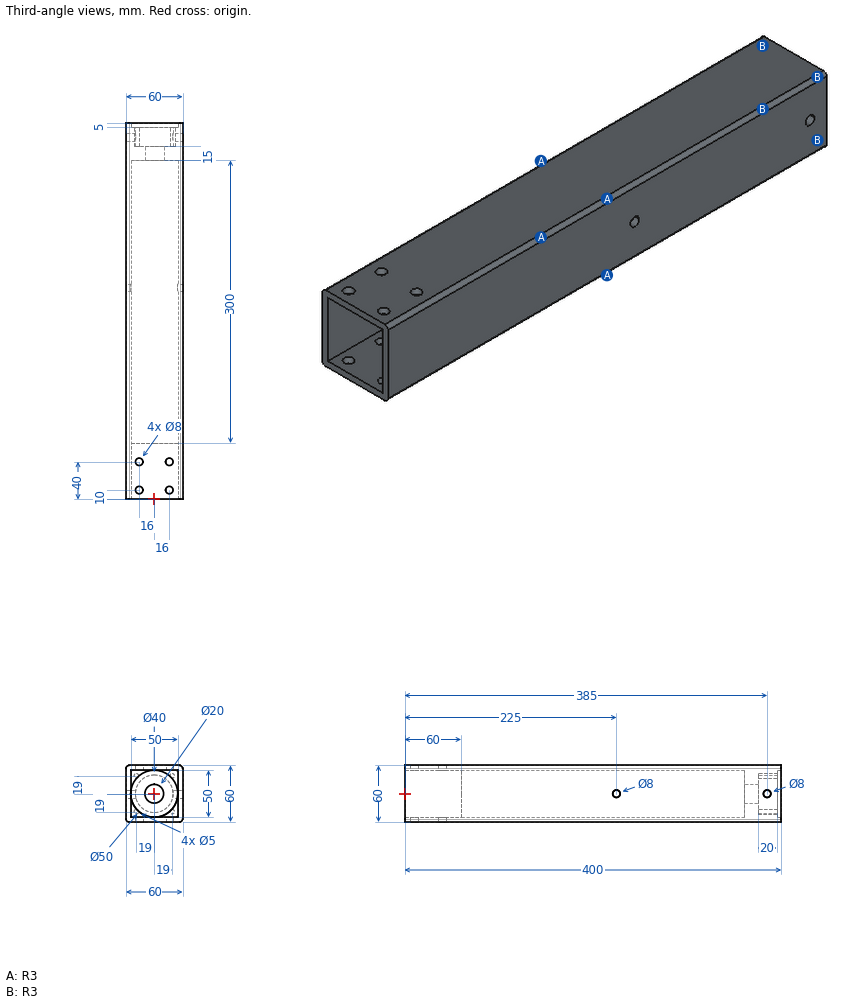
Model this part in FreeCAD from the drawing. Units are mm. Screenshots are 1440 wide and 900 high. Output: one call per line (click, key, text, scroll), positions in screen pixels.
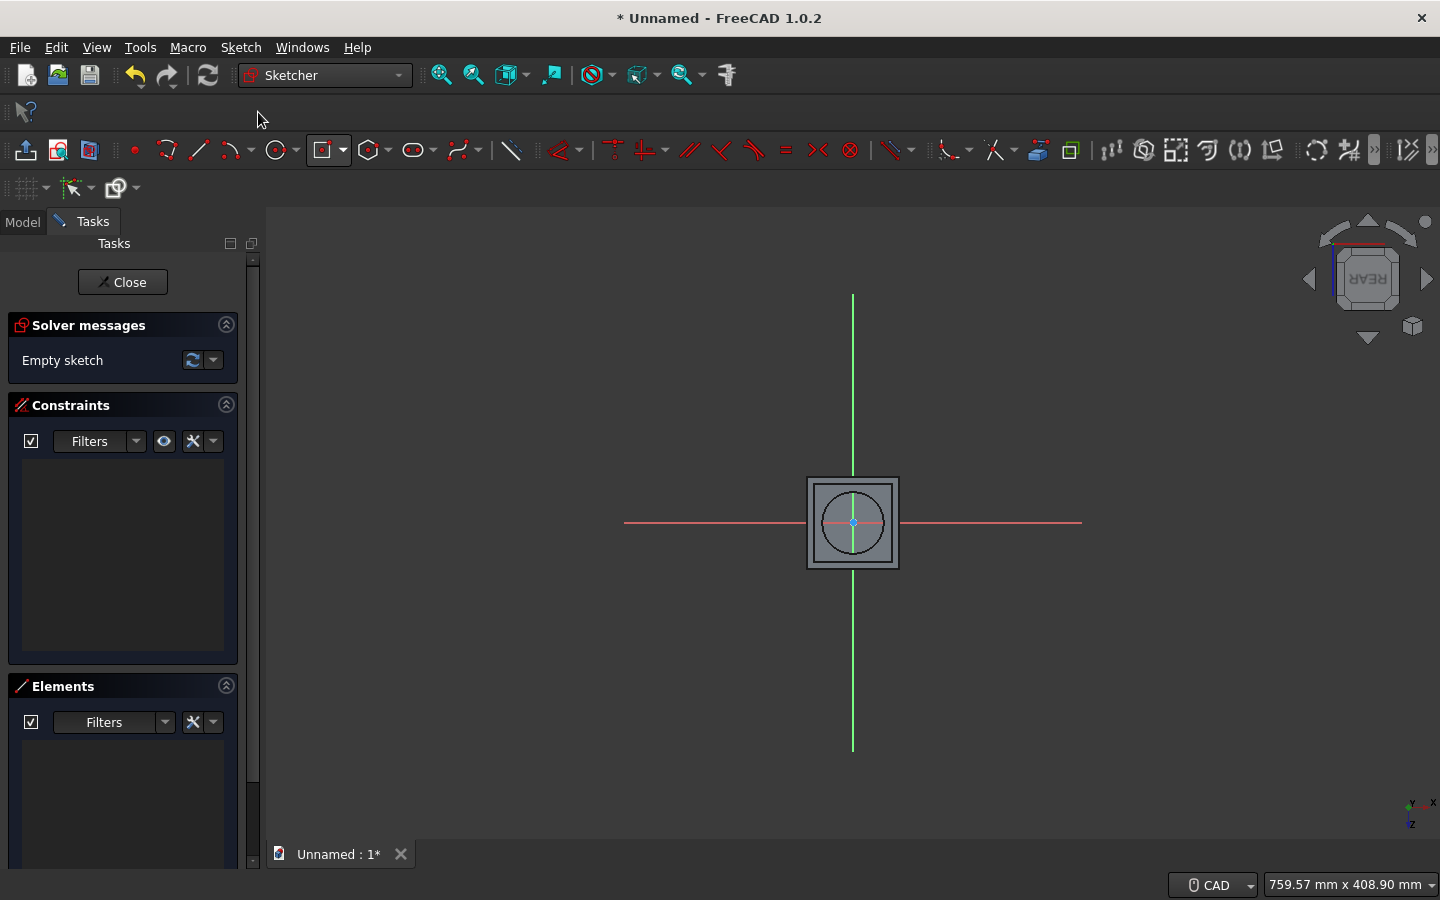
scroll(858, 523, up, 13)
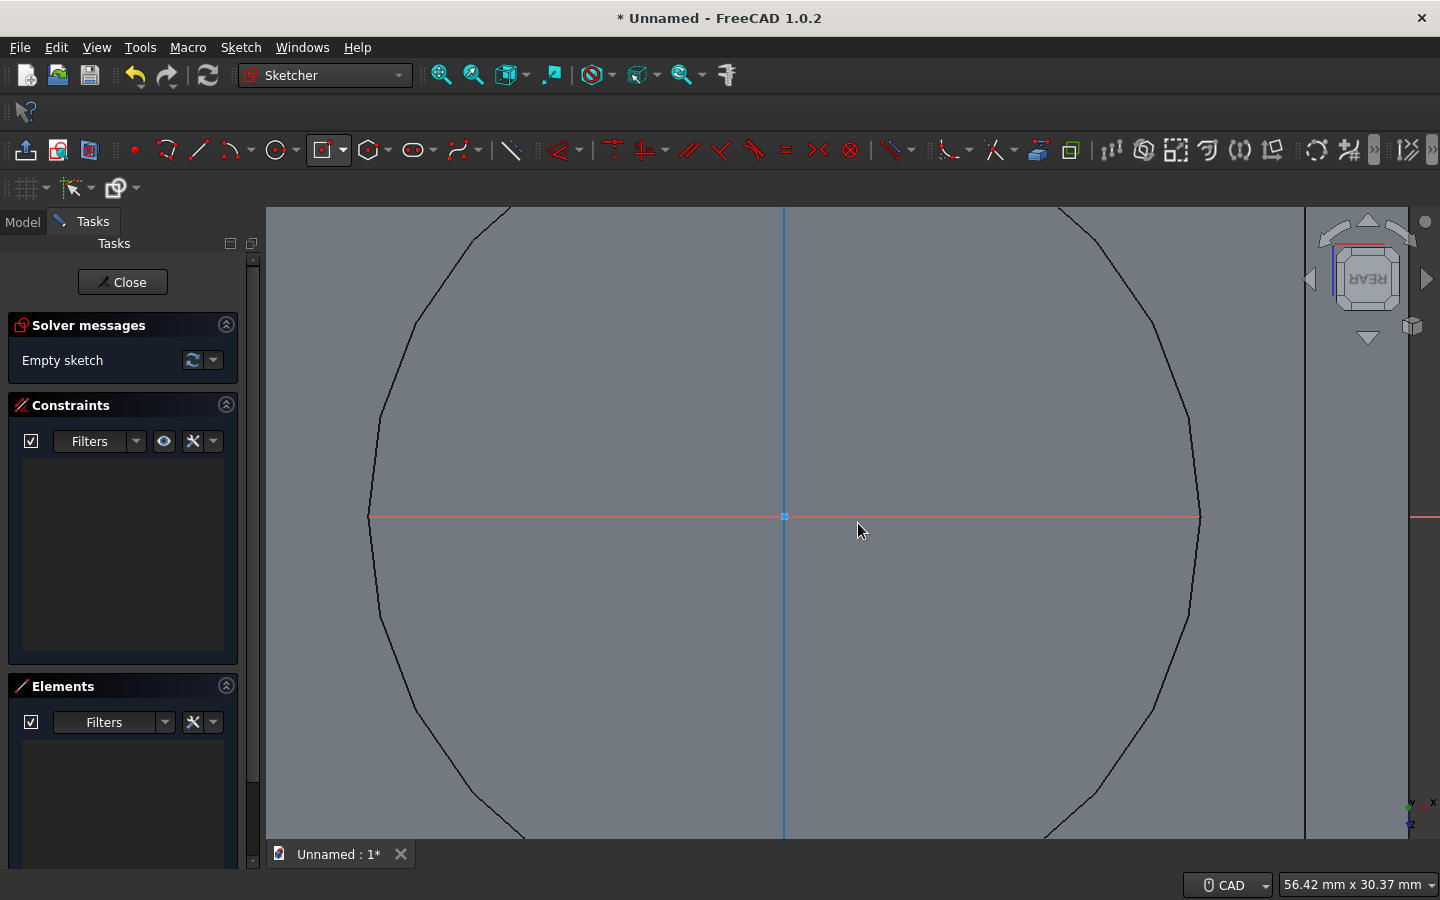
key(g)
key(c)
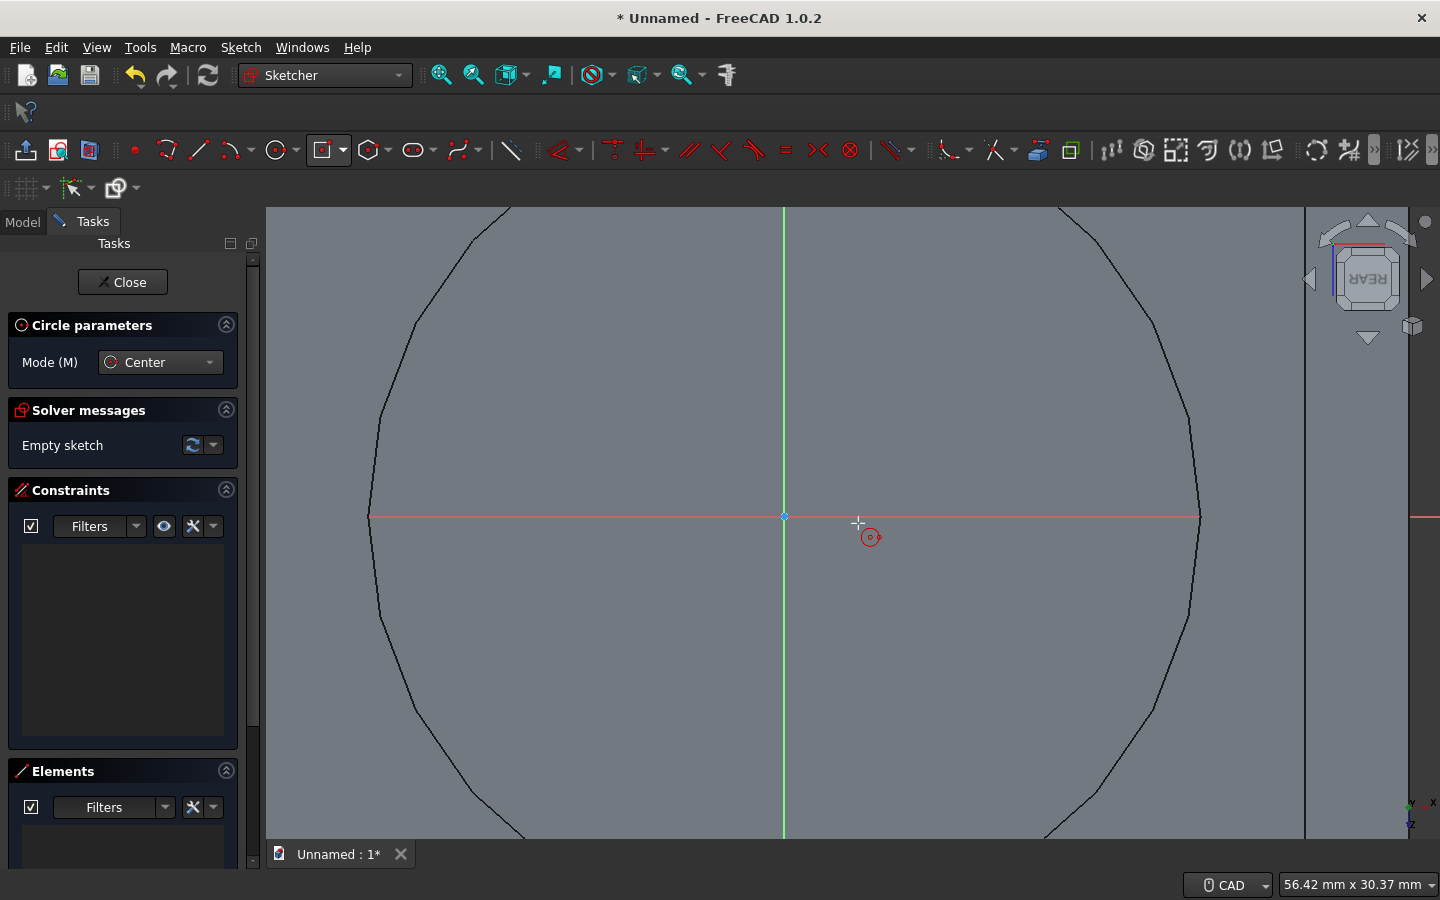
click(784, 517)
move(932, 370)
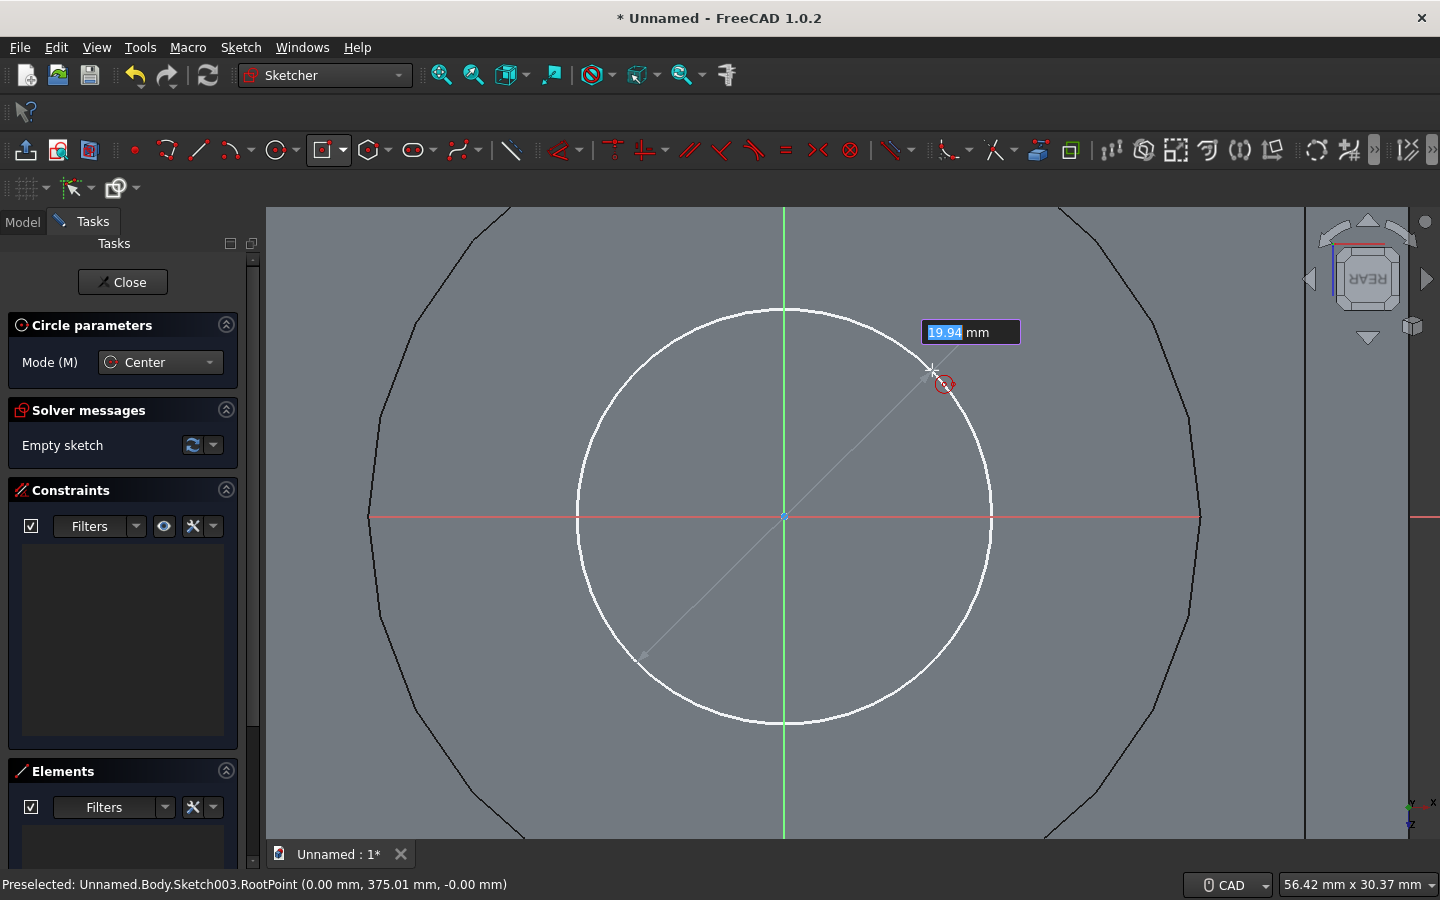
text(20)
key(Return)
key(Escape)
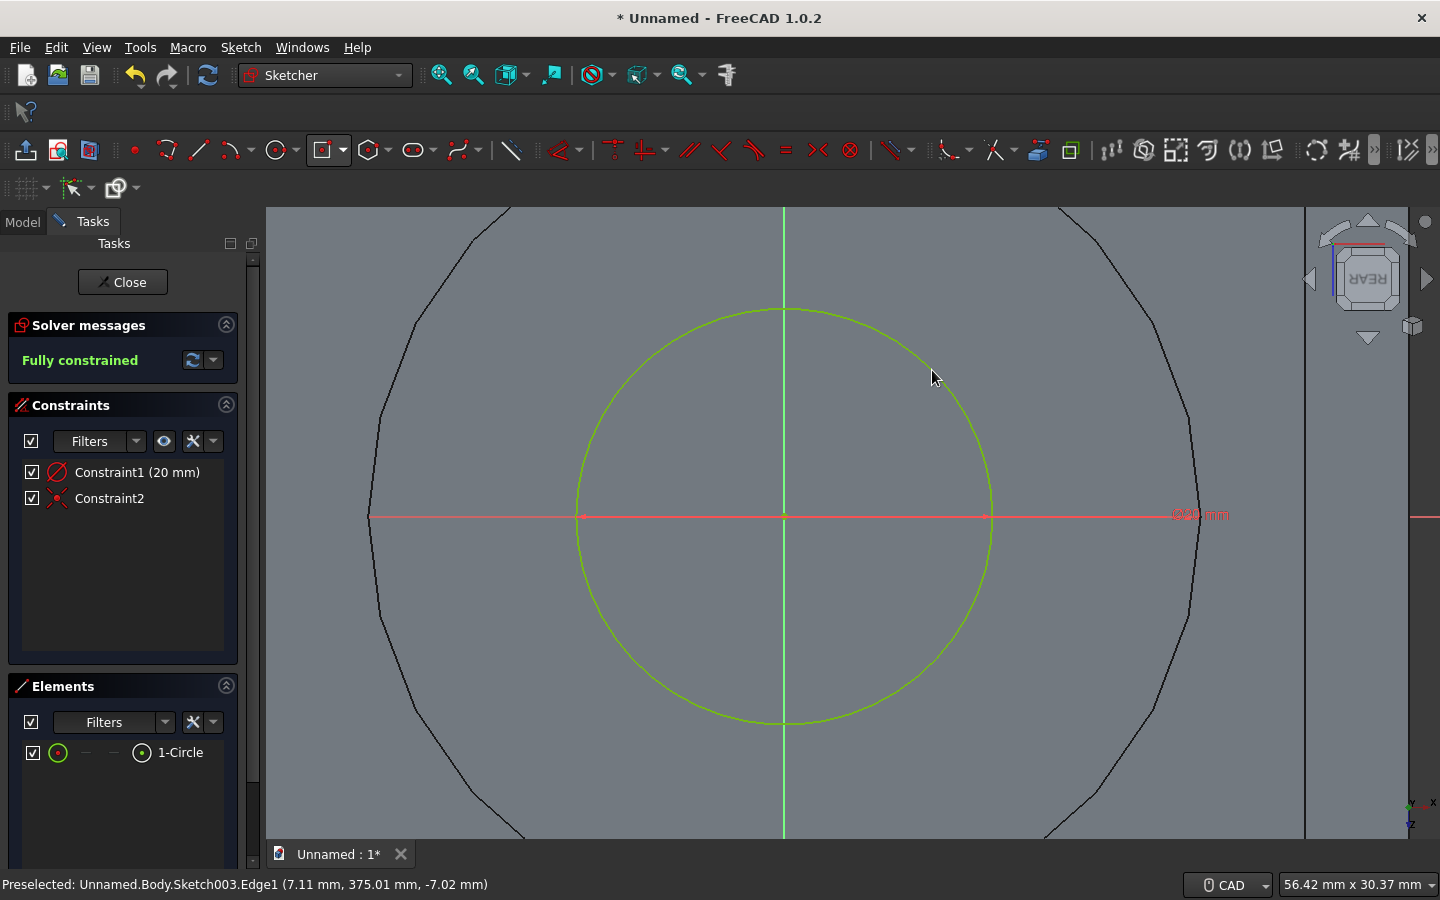
click(123, 282)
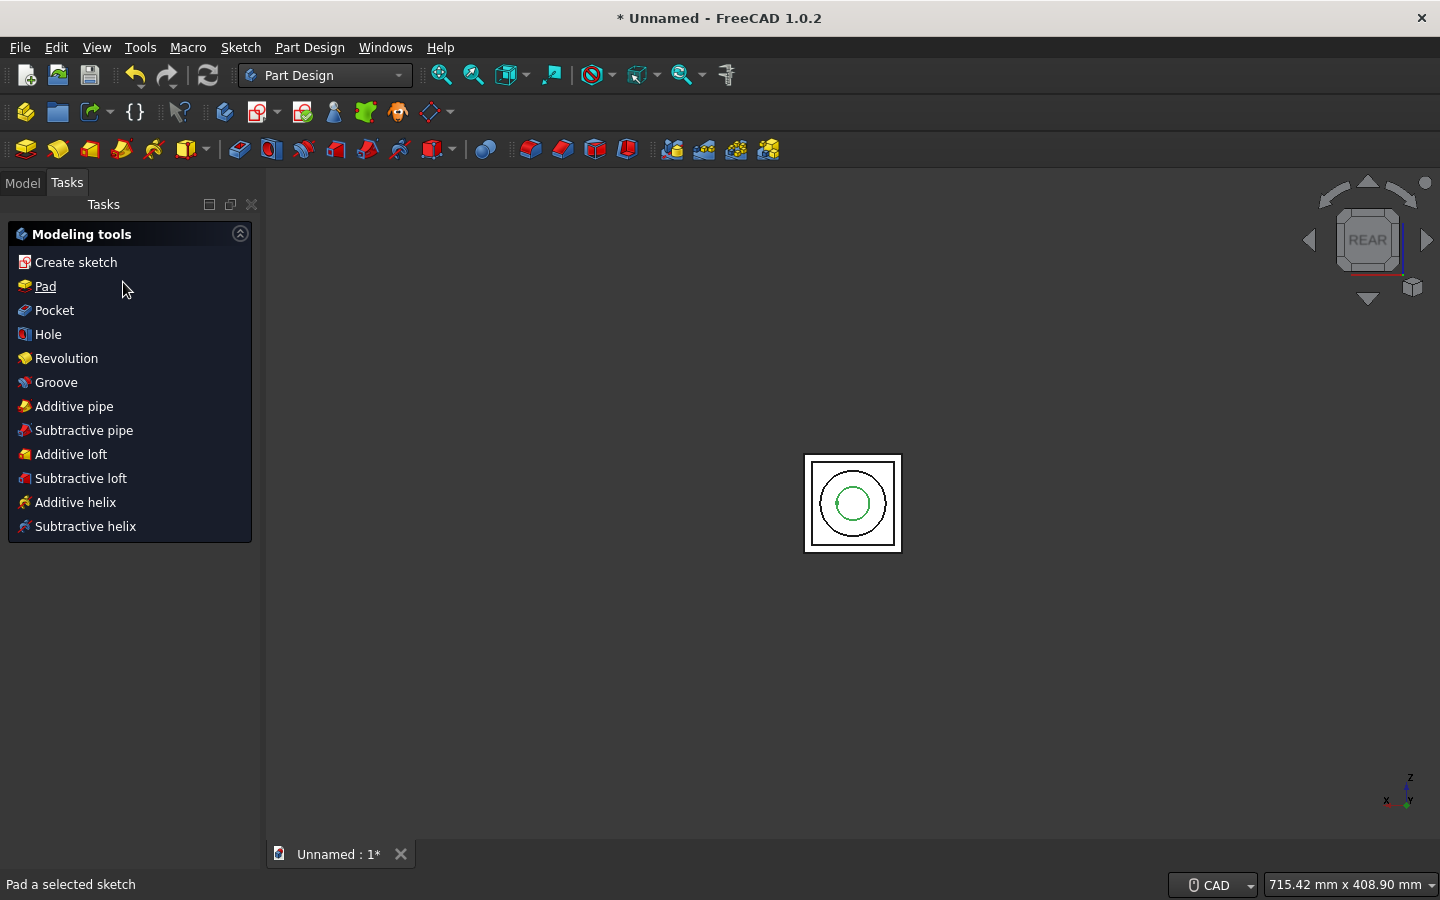
click(240, 150)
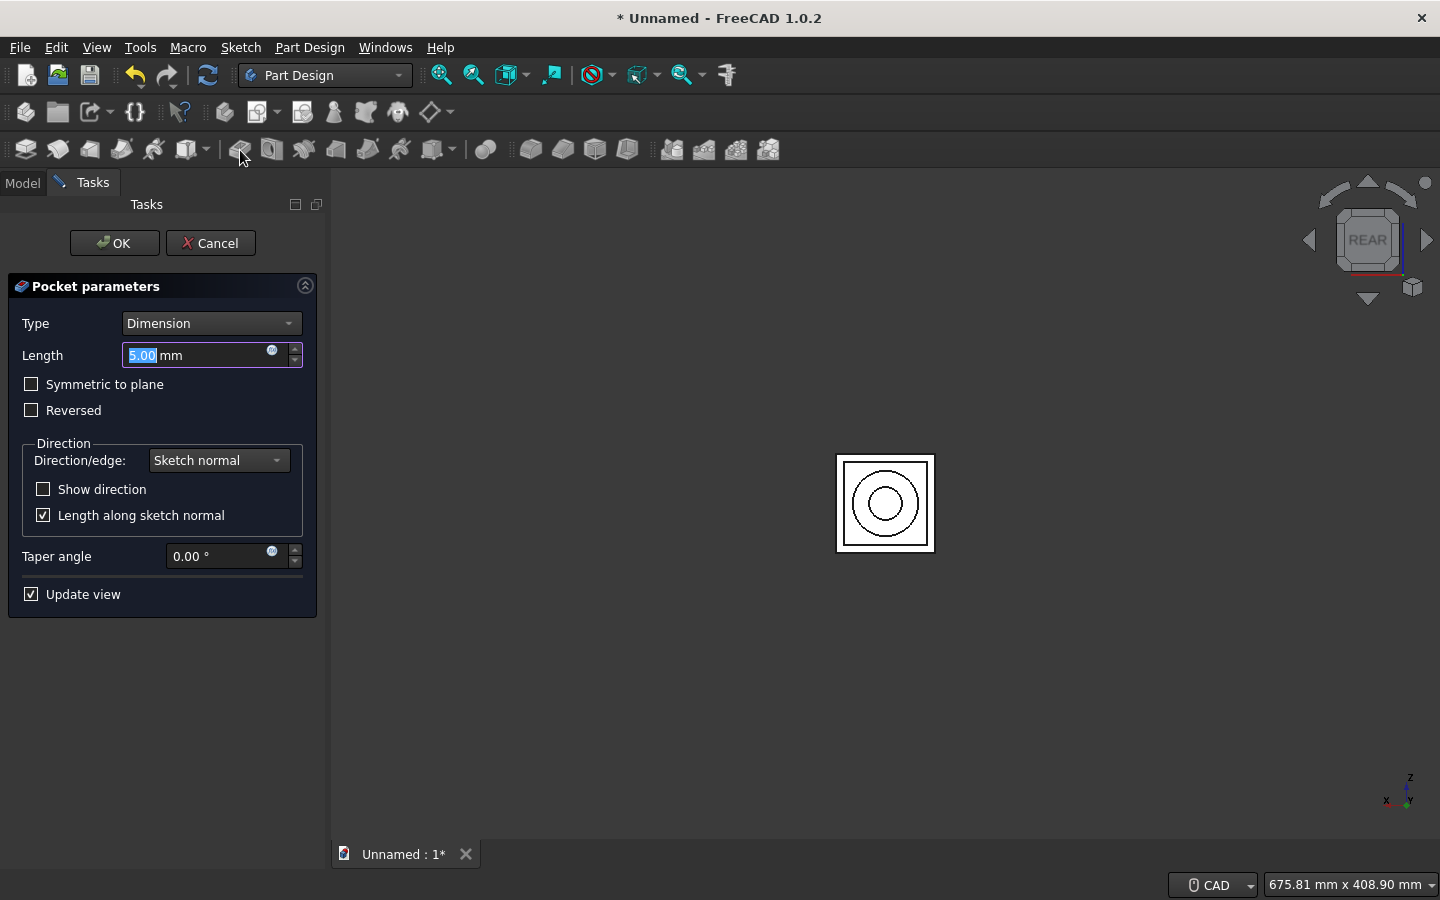
text(15)
key(Tab)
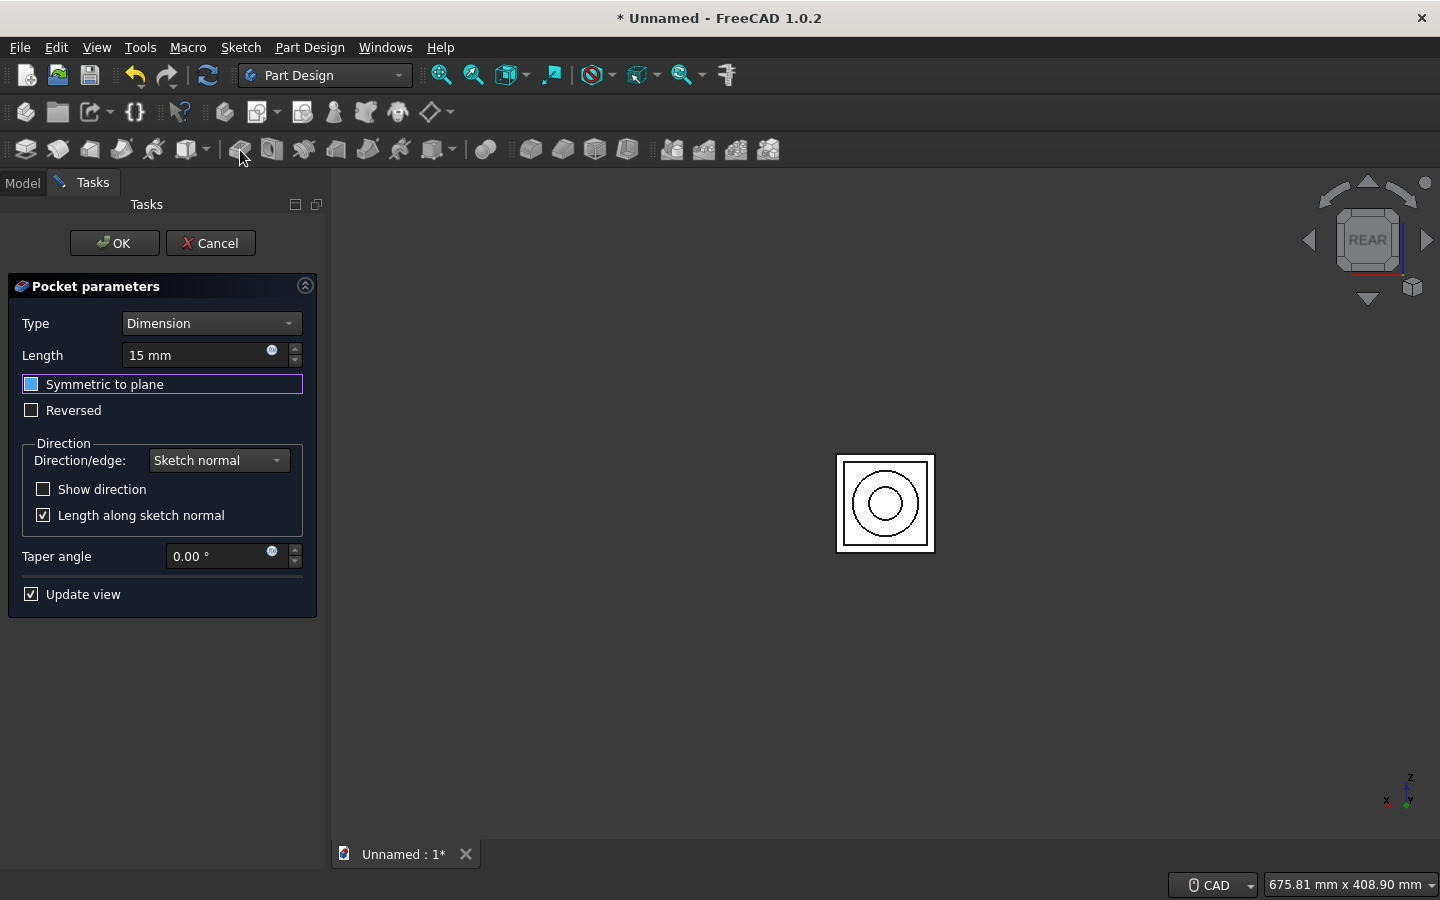
click(115, 243)